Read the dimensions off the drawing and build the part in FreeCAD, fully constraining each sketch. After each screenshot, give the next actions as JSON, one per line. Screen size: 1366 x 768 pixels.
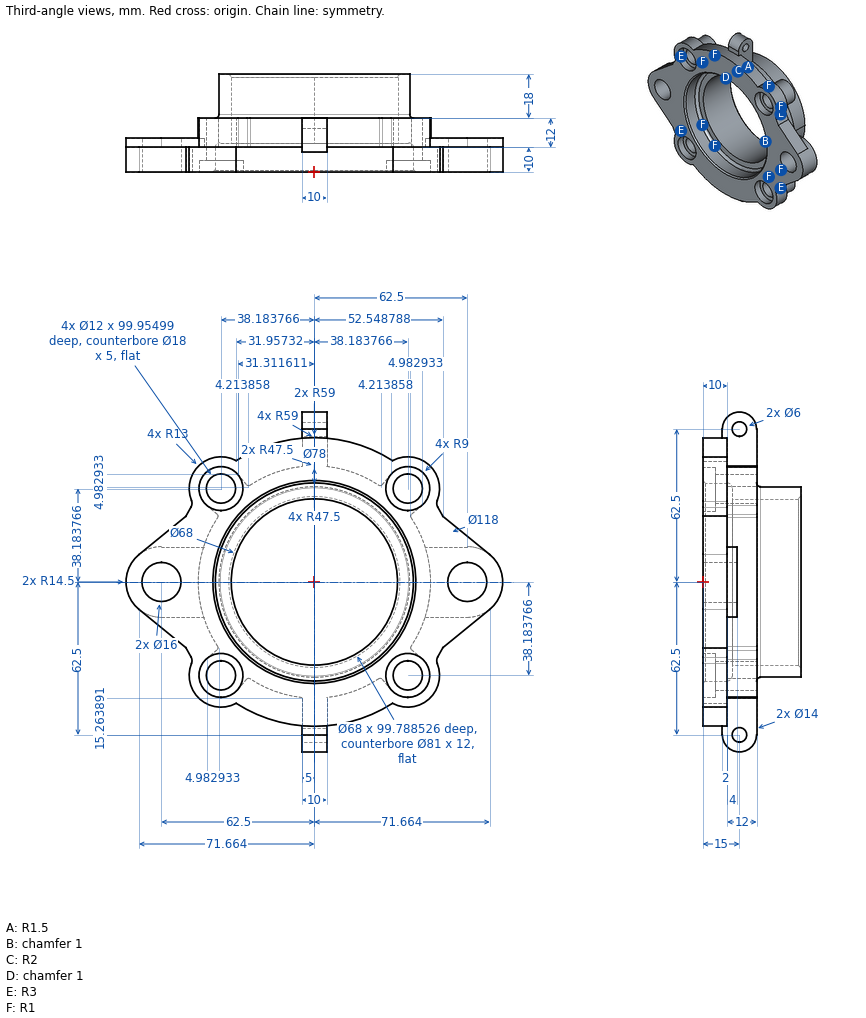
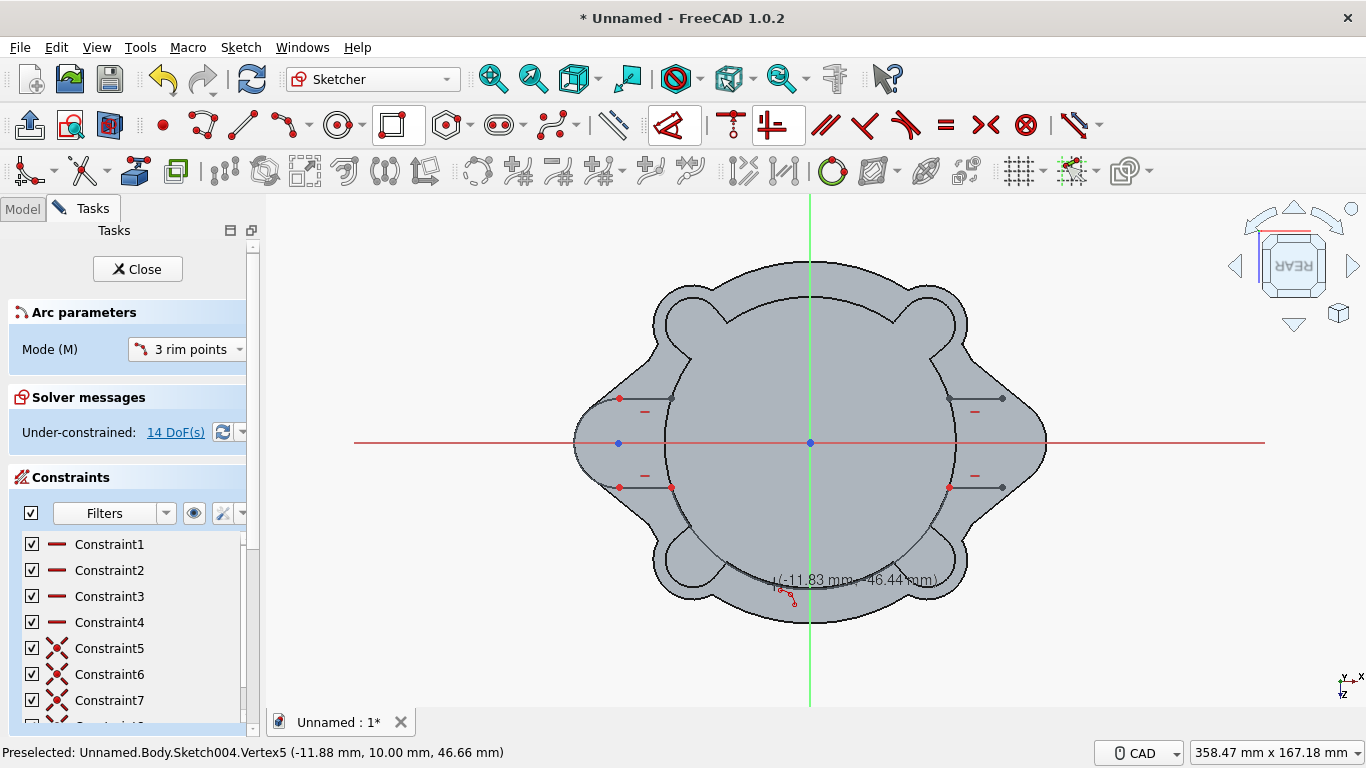
{"action": "left_click", "coordinate": [1002, 488]}
{"action": "left_click", "coordinate": [1002, 399]}
{"action": "left_click", "coordinate": [1038, 469]}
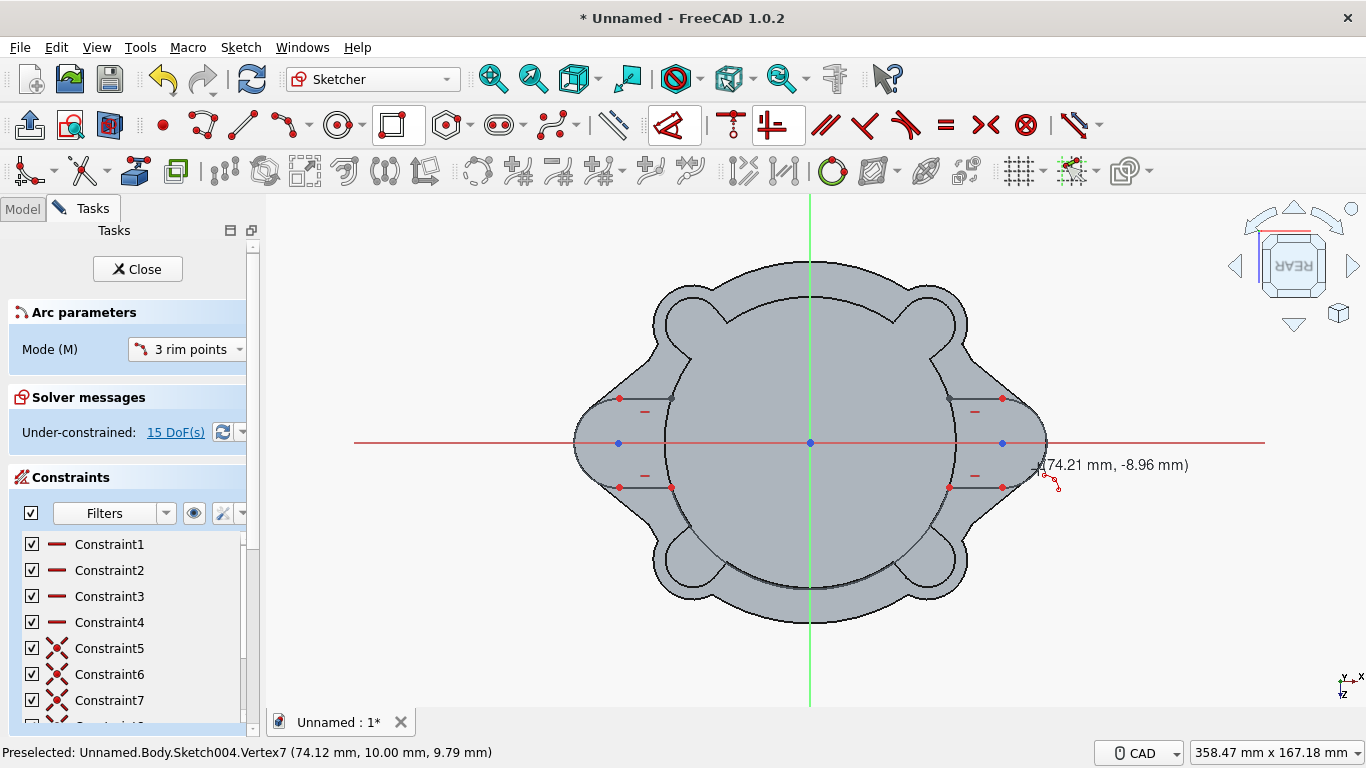
{"action": "left_click", "coordinate": [949, 399]}
{"action": "left_click", "coordinate": [671, 399]}
{"action": "left_click", "coordinate": [847, 301]}
{"action": "key", "text": "Escape"}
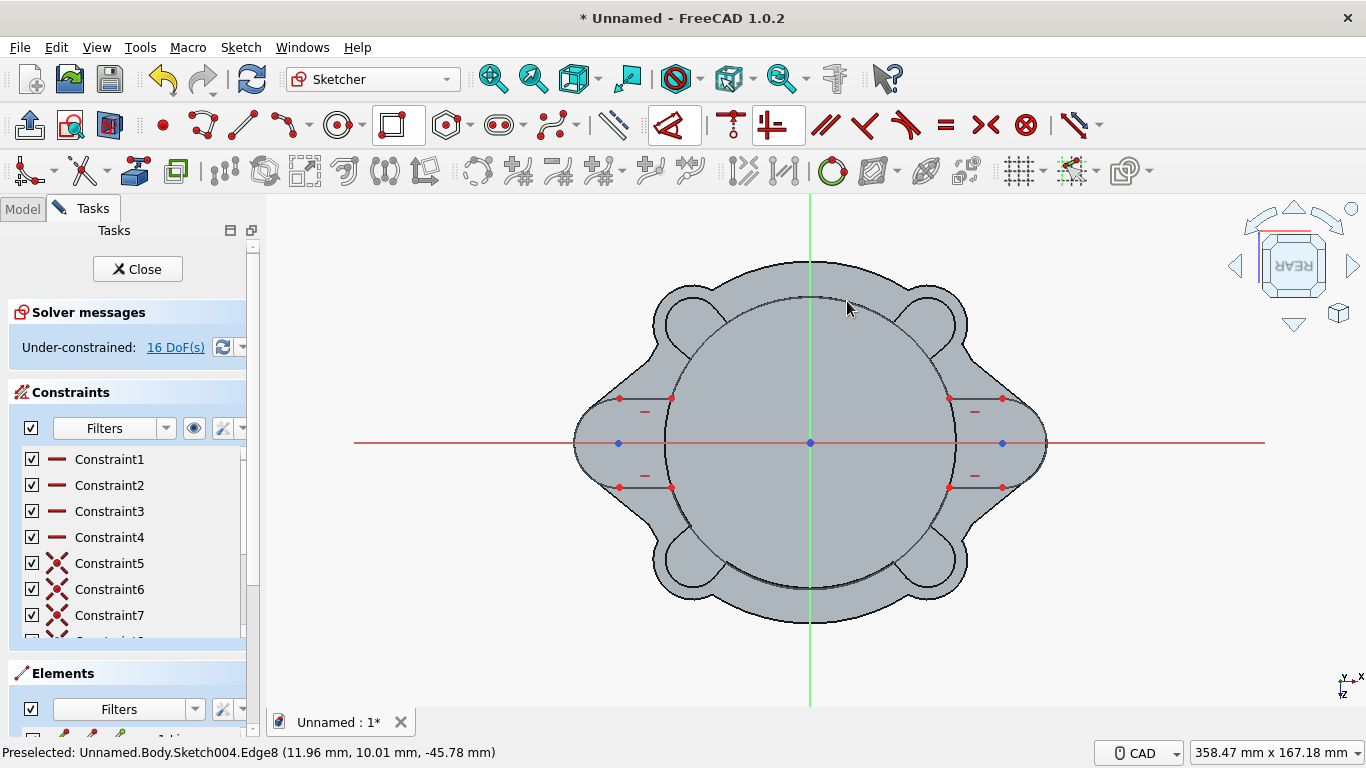
{"action": "left_click", "coordinate": [655, 399]}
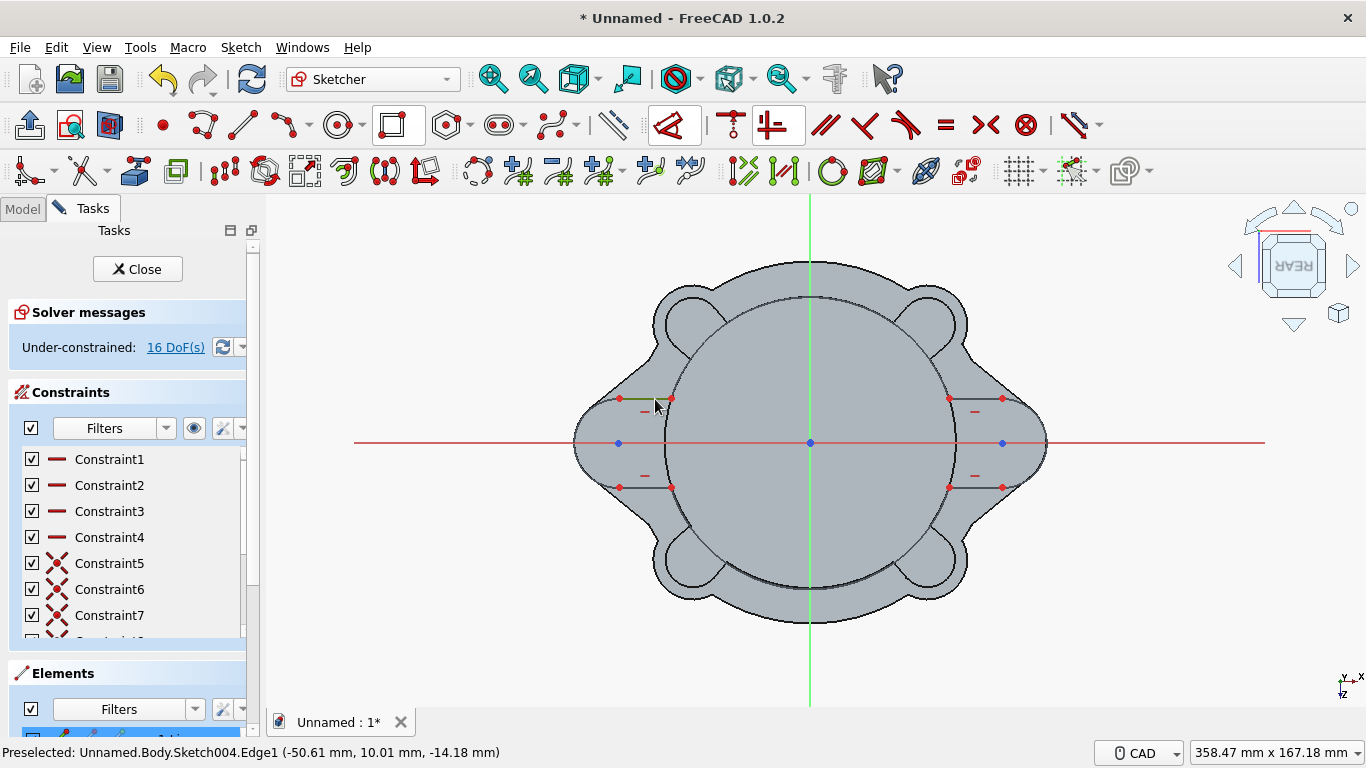
{"action": "left_click", "coordinate": [583, 417]}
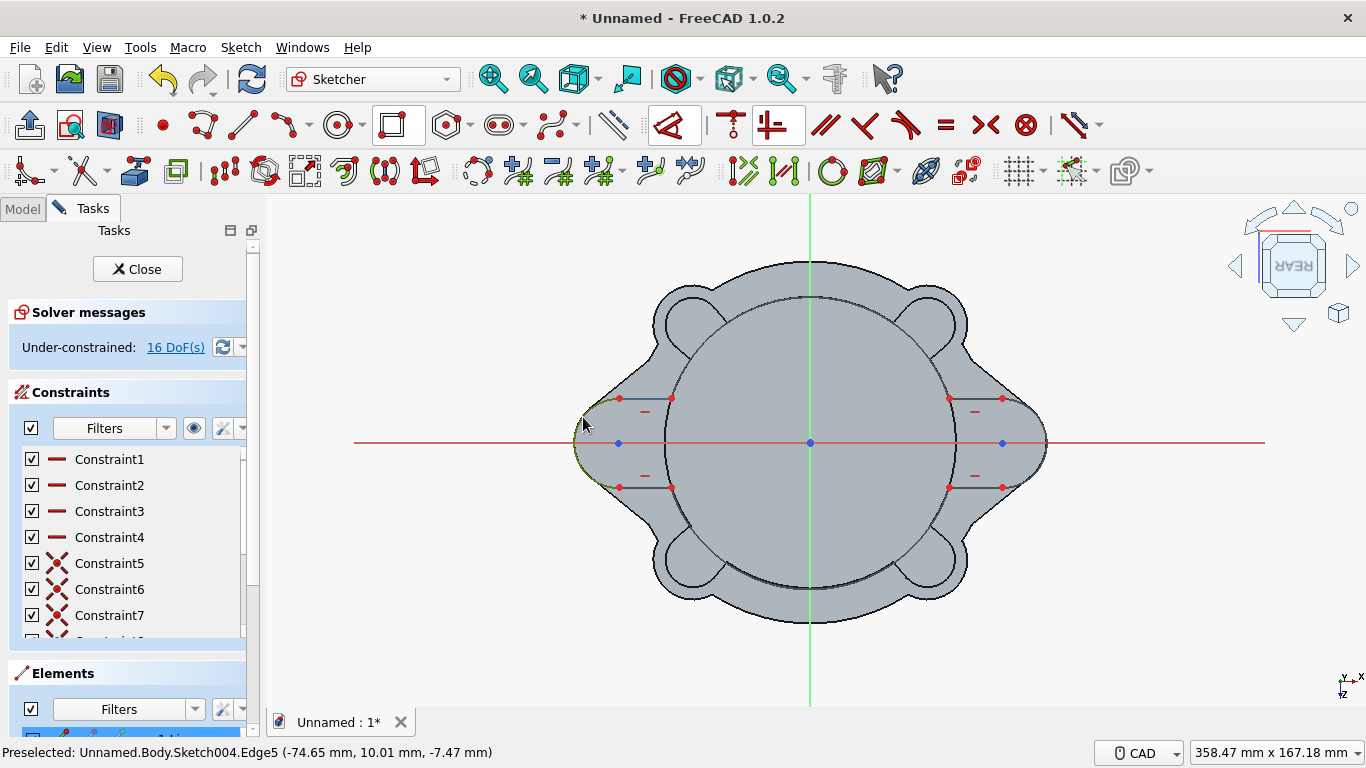
{"action": "left_click", "coordinate": [906, 126]}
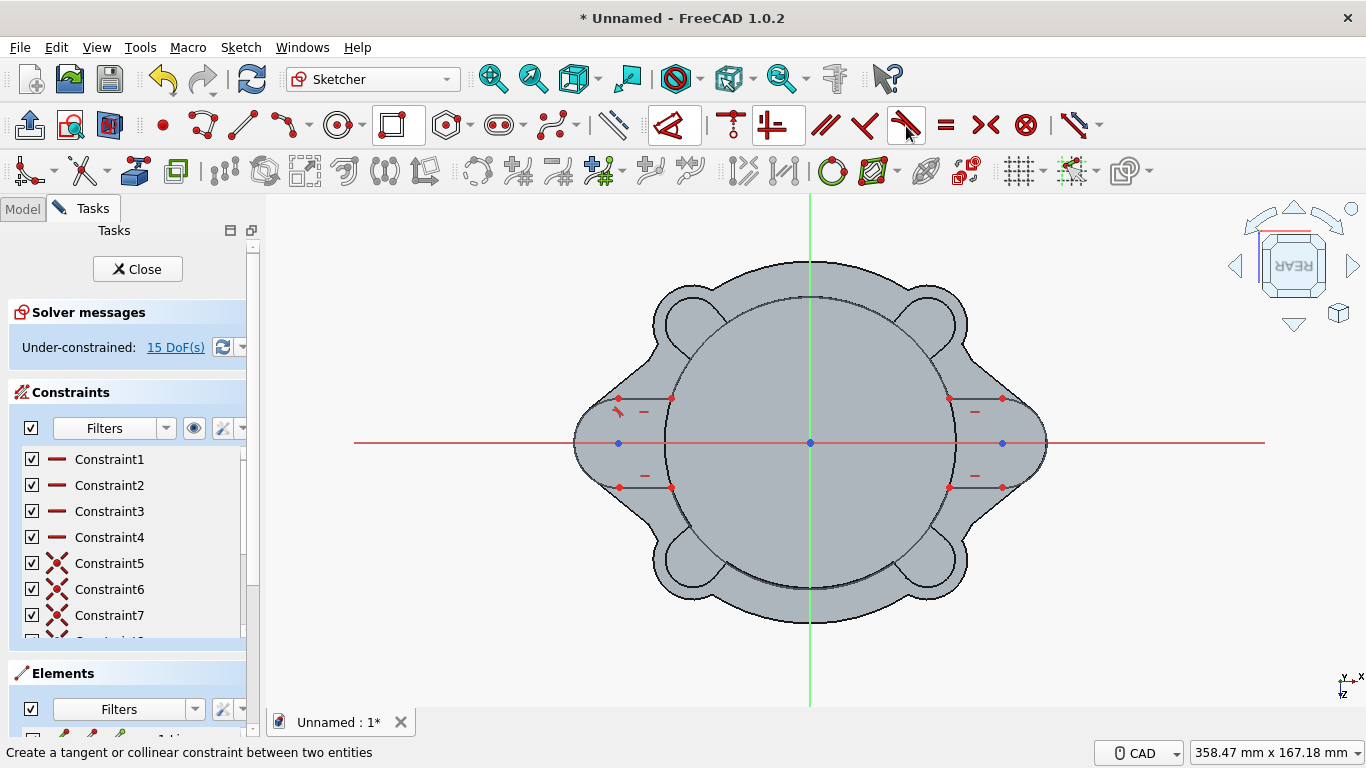
{"action": "left_click", "coordinate": [635, 488]}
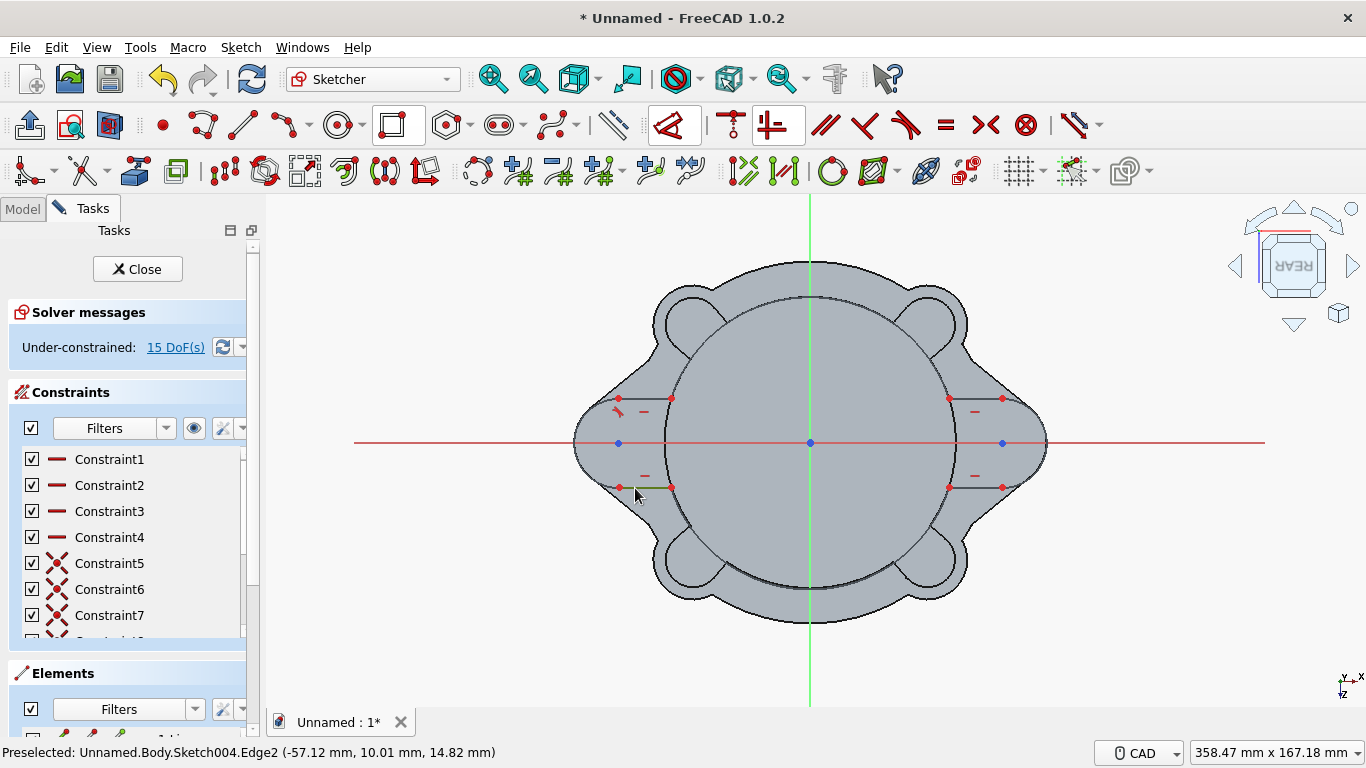
{"action": "left_click", "coordinate": [583, 417]}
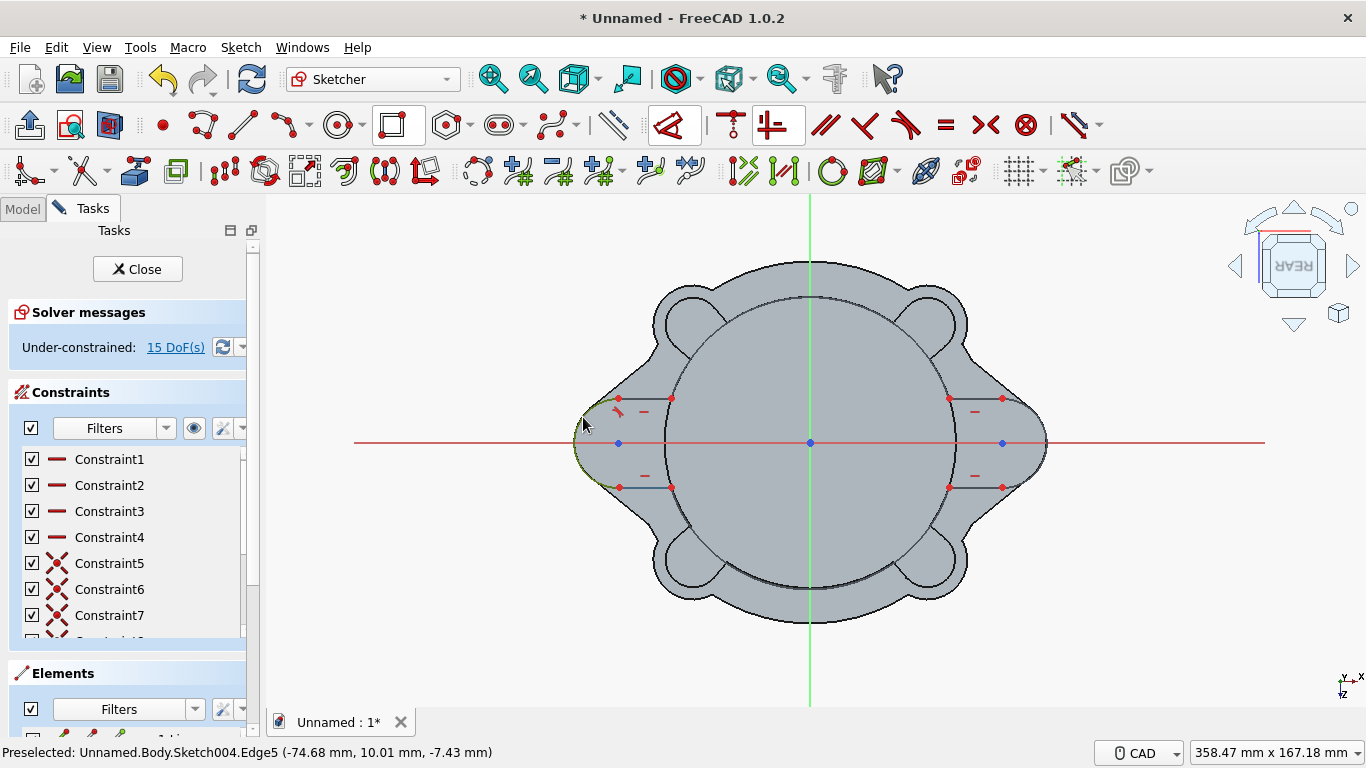
{"action": "left_click", "coordinate": [906, 126]}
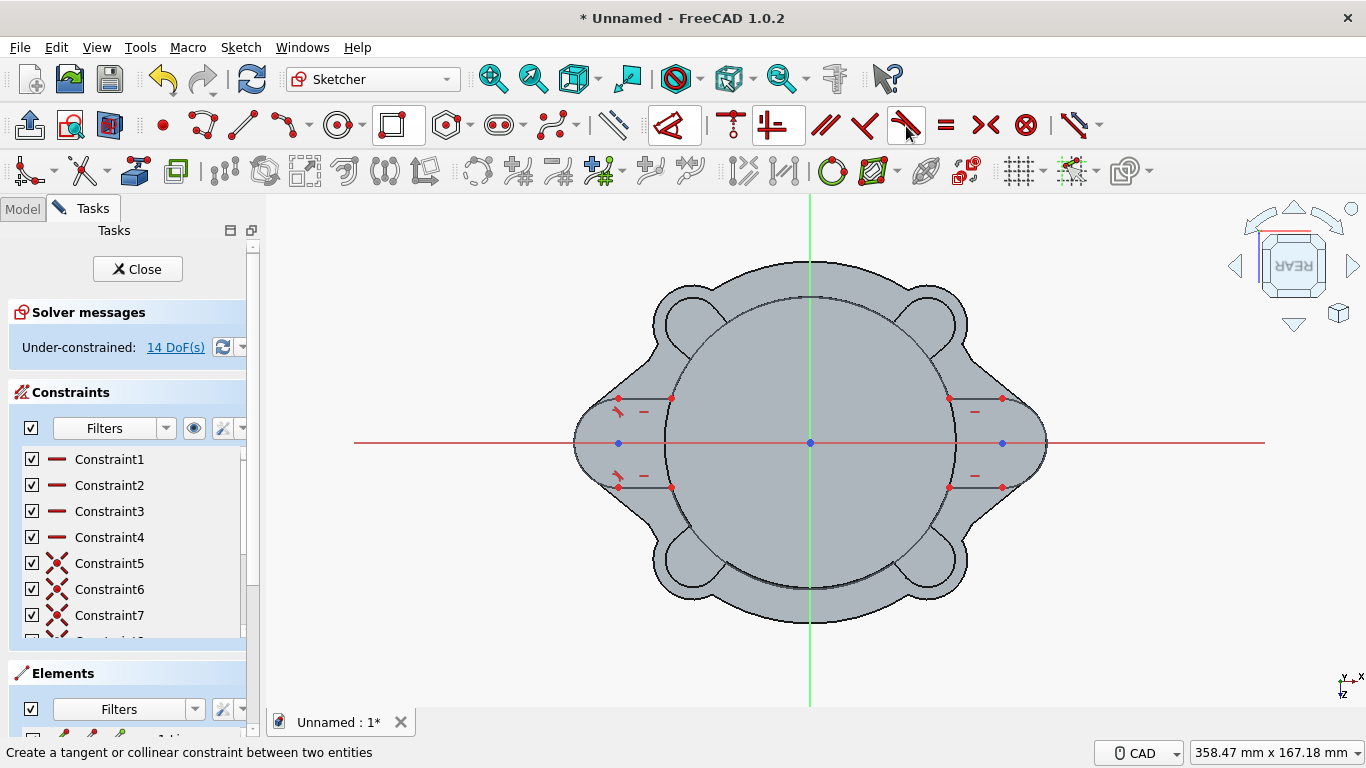
{"action": "left_click", "coordinate": [965, 488]}